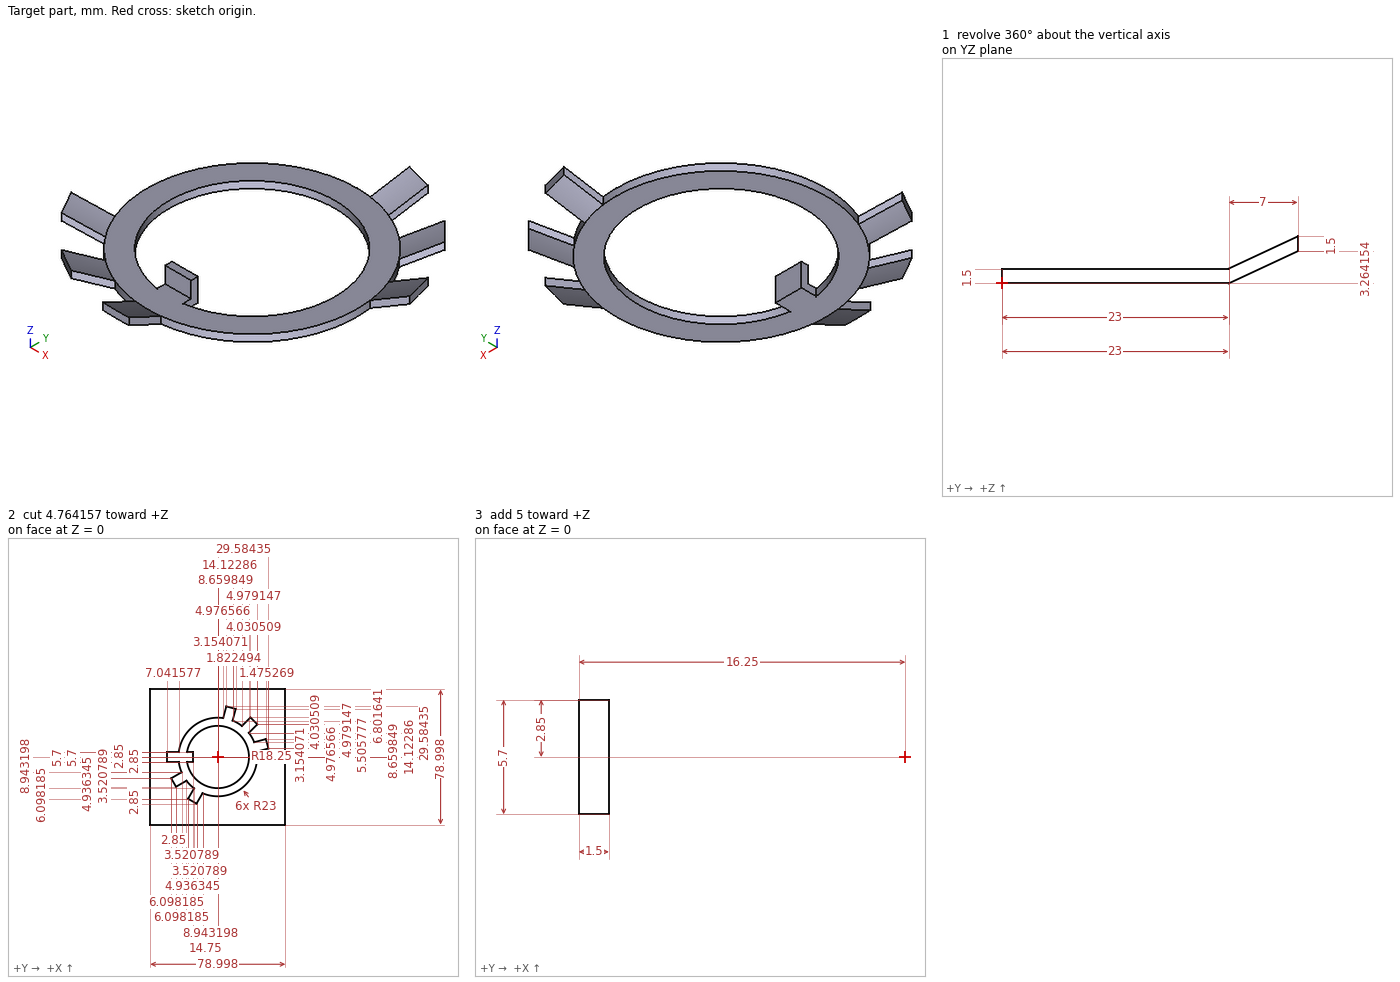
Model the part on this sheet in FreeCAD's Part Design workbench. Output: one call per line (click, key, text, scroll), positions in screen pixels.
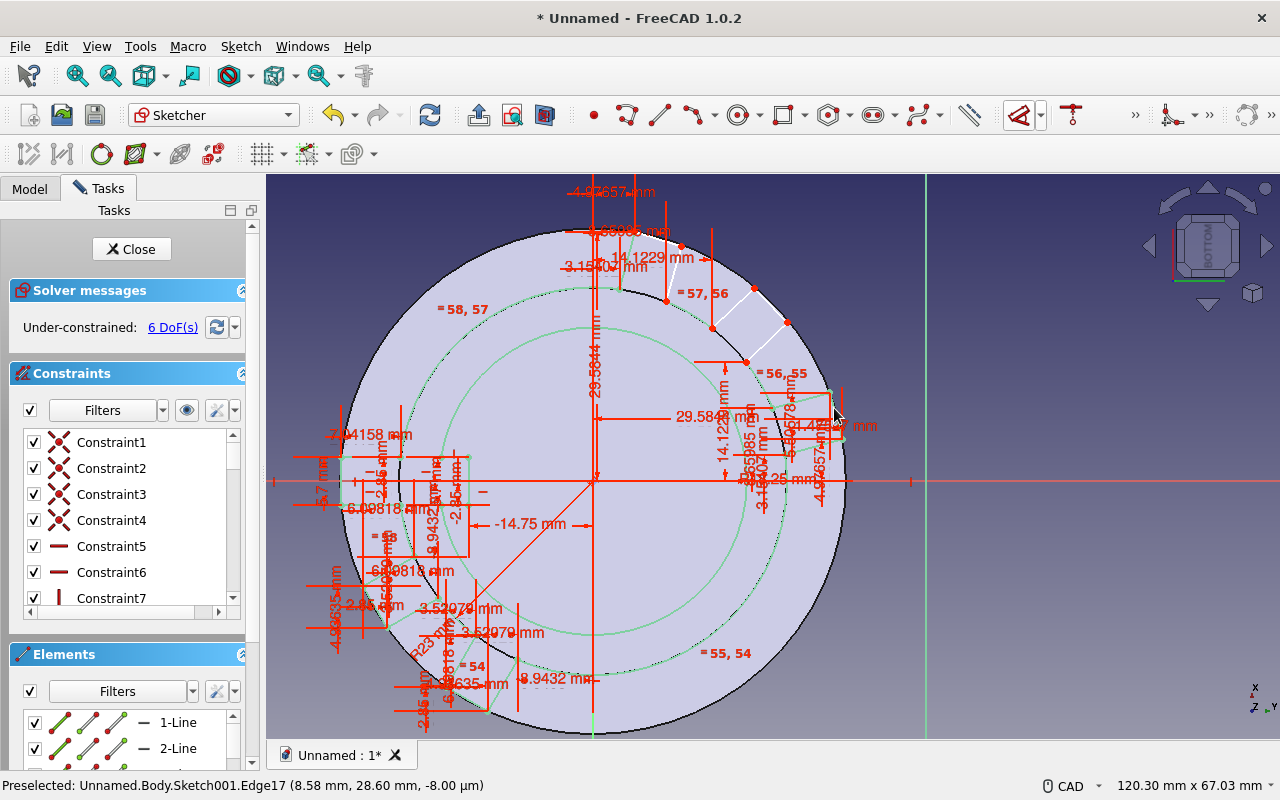
click(758, 350)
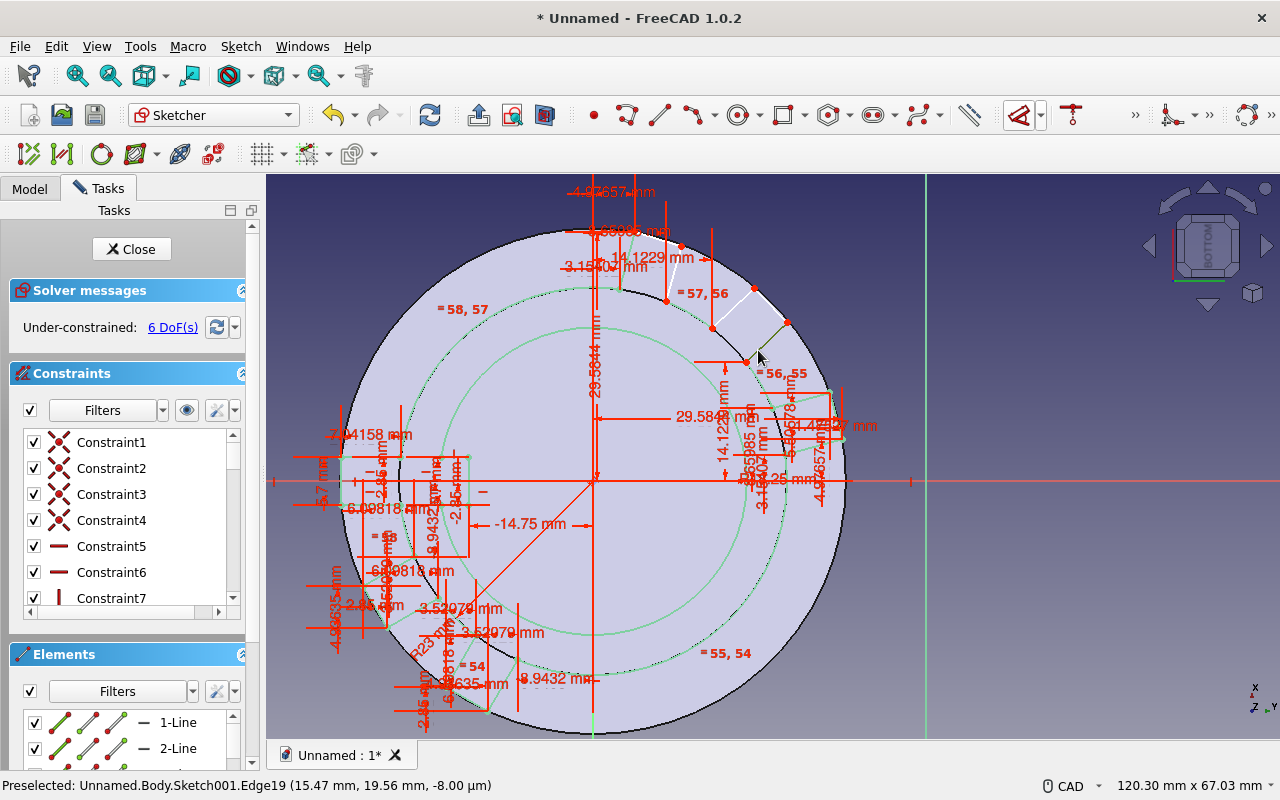
key(l)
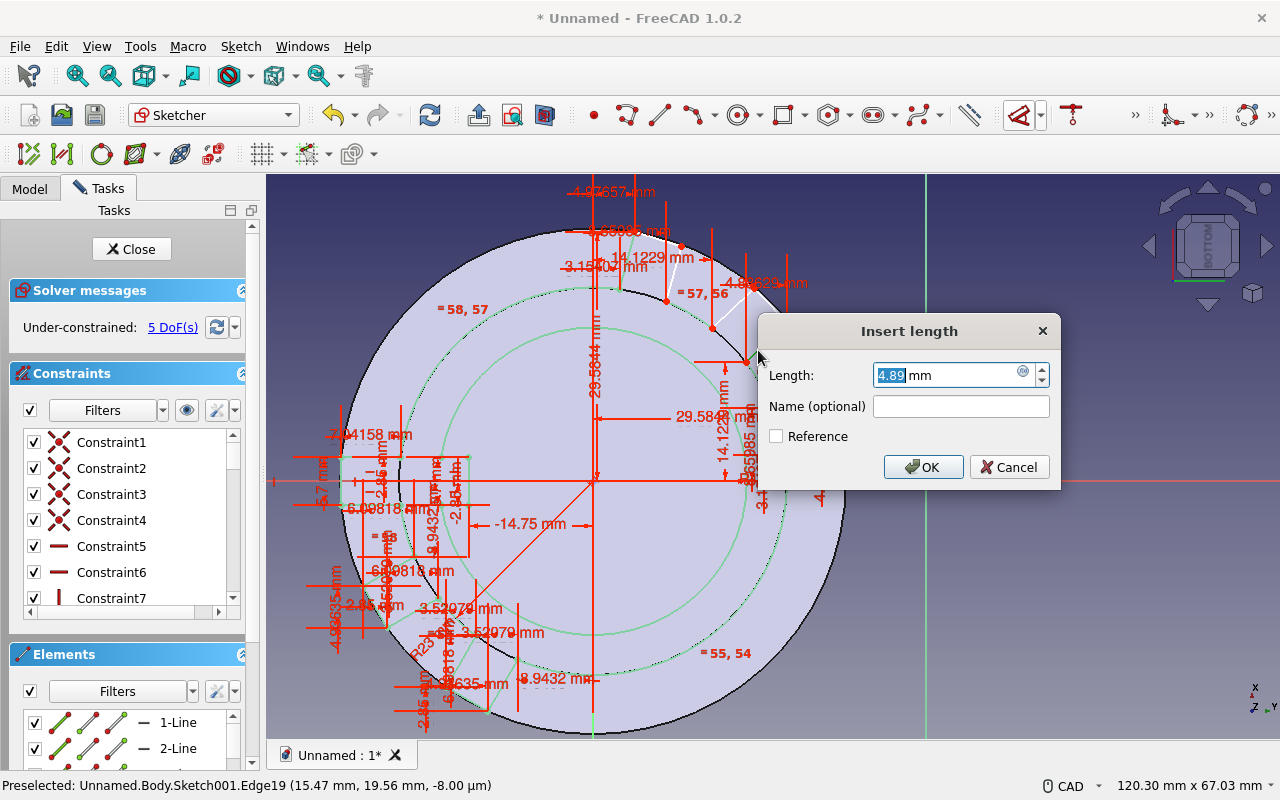
text(4.979147)
key(Return)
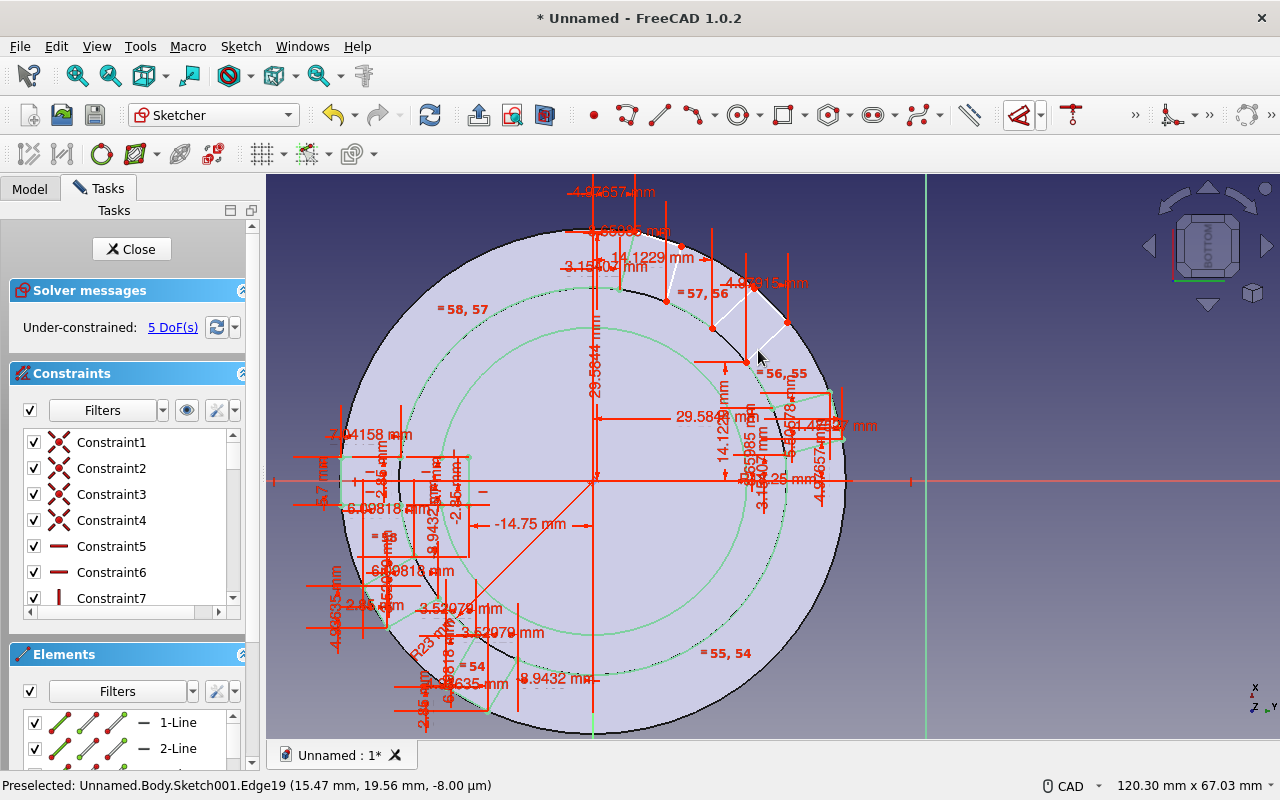
click(759, 350)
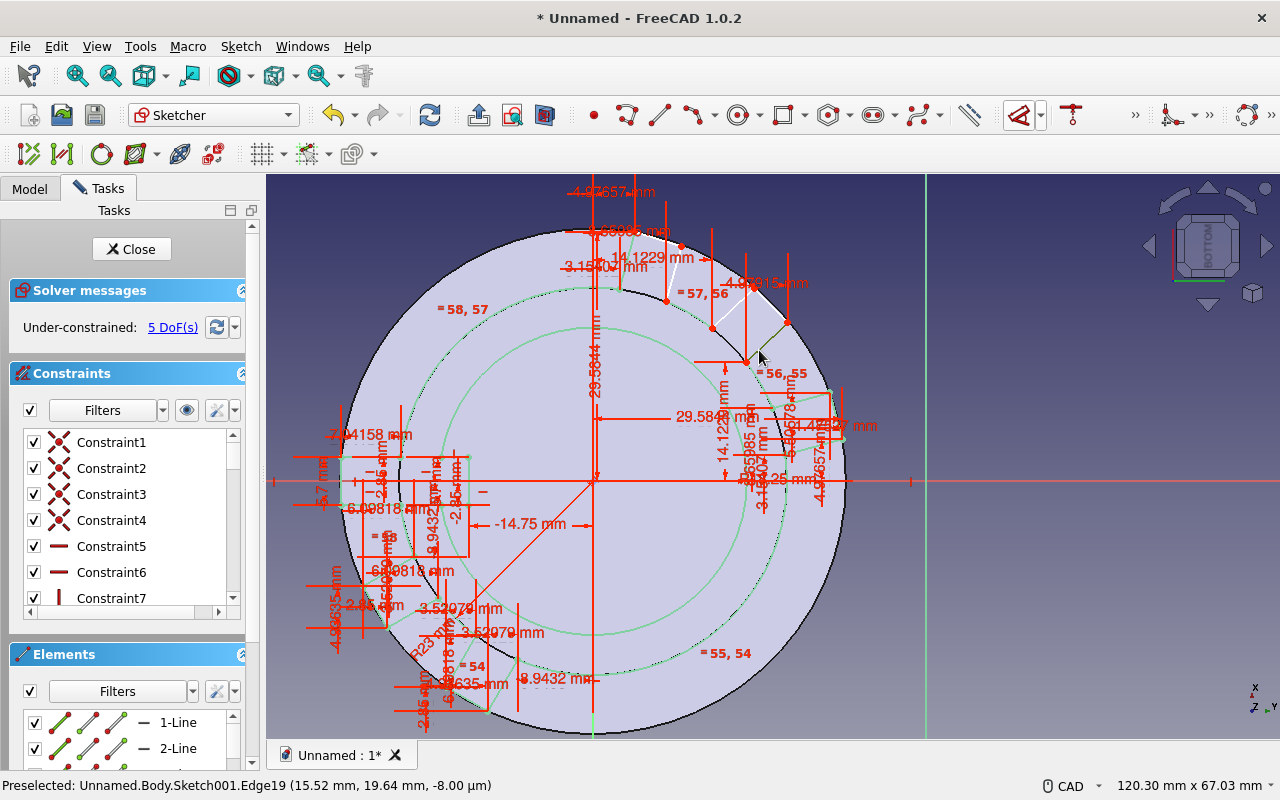
key(i)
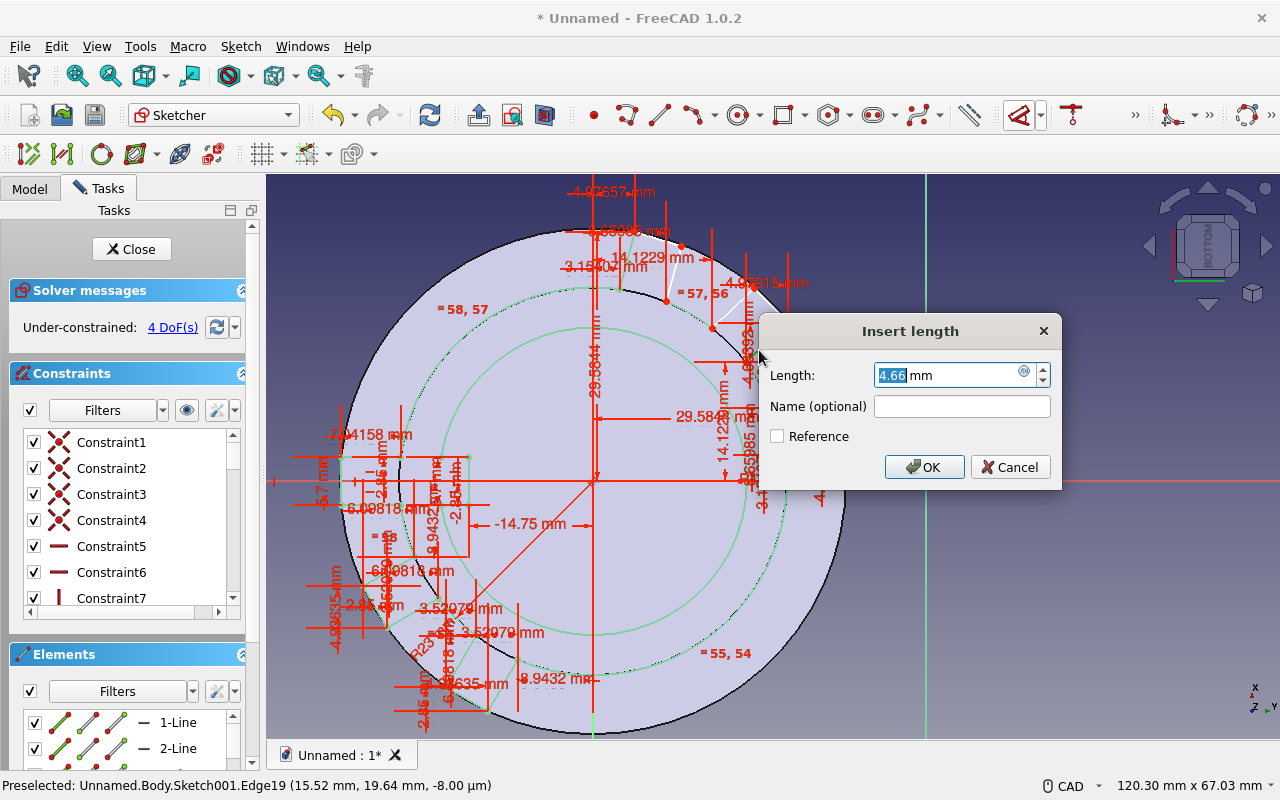
text(4.979147)
key(Return)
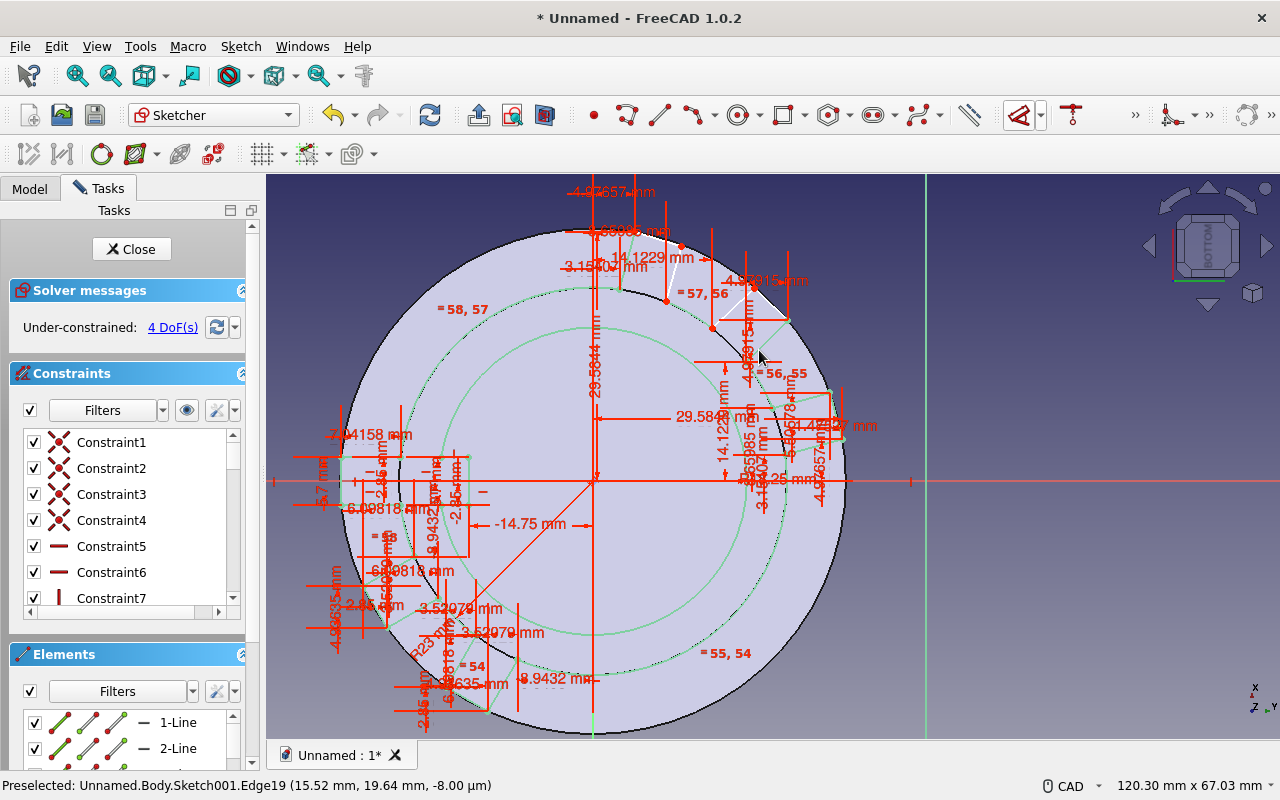
click(778, 311)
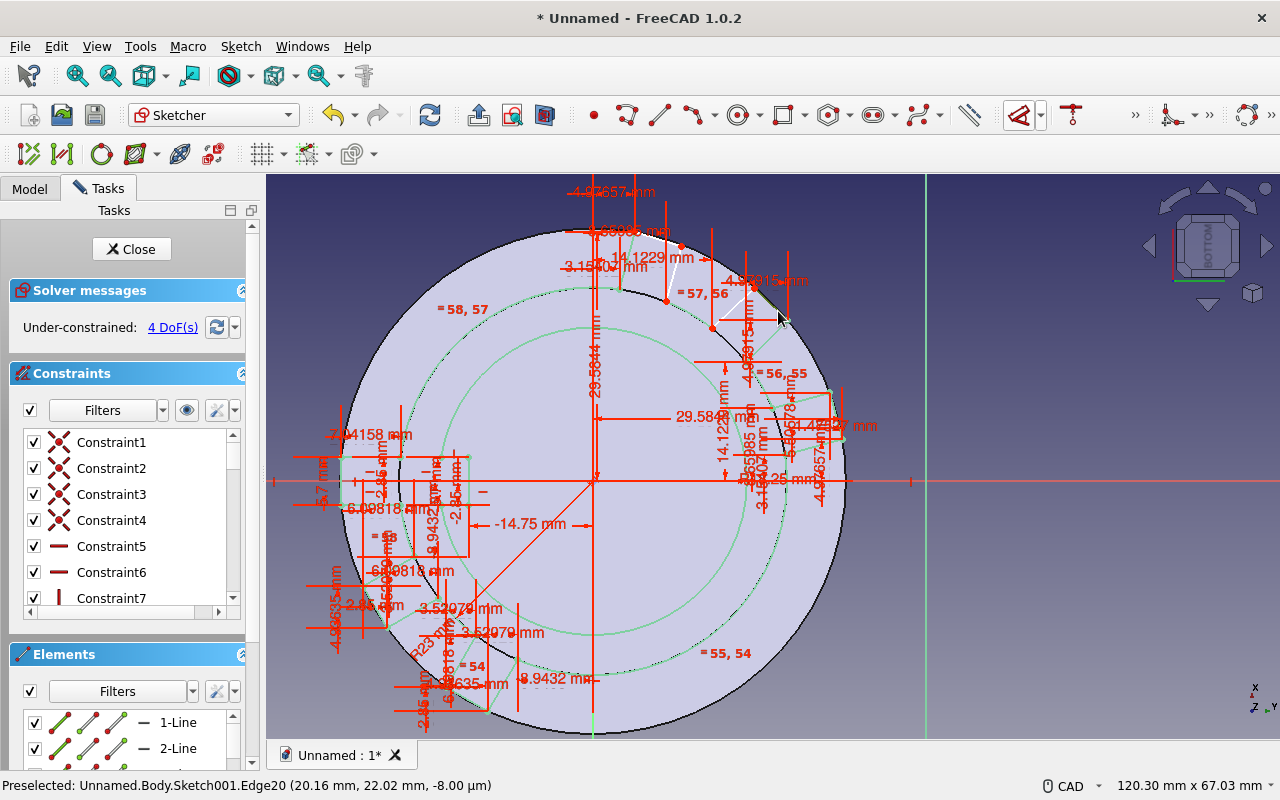
key(l)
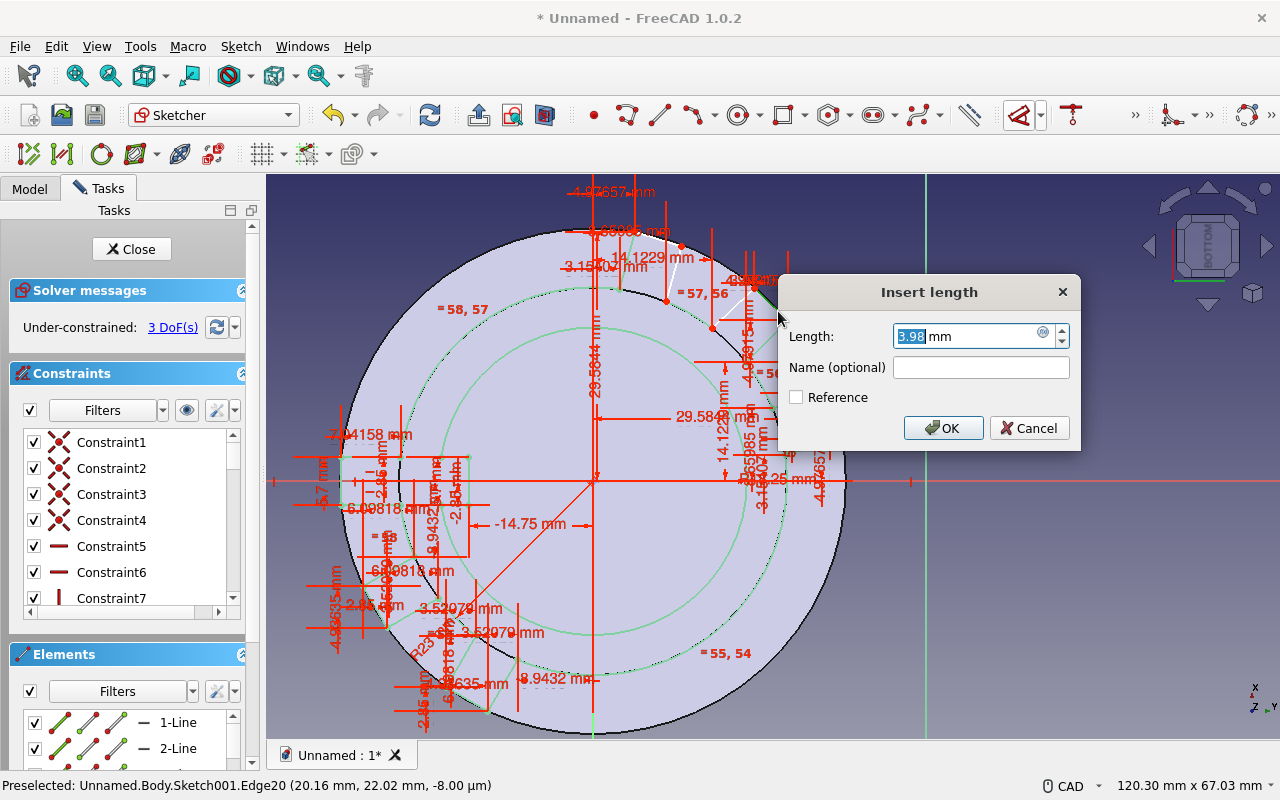
text(4.030509)
key(Return)